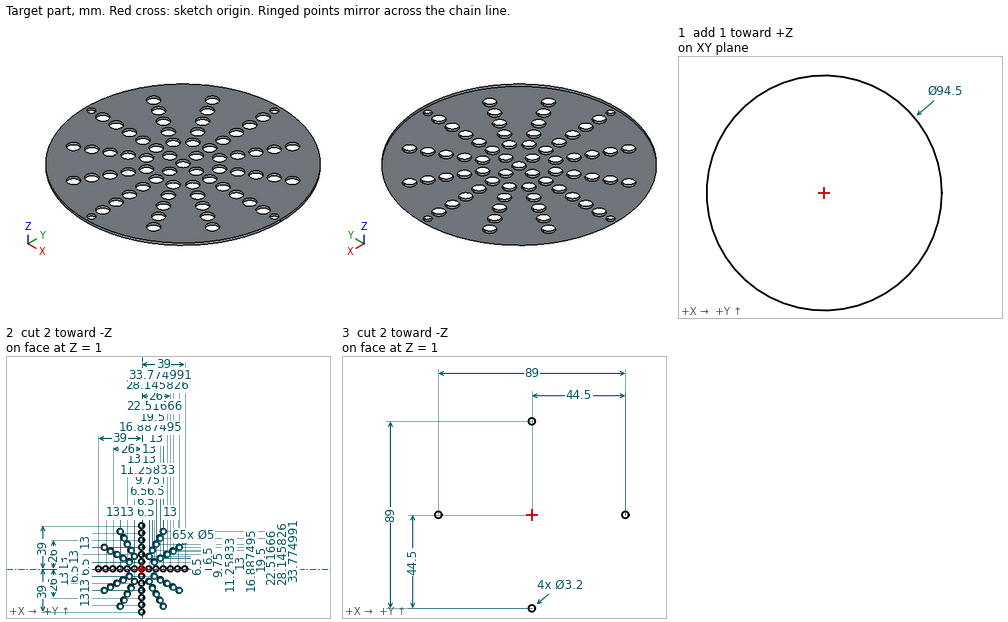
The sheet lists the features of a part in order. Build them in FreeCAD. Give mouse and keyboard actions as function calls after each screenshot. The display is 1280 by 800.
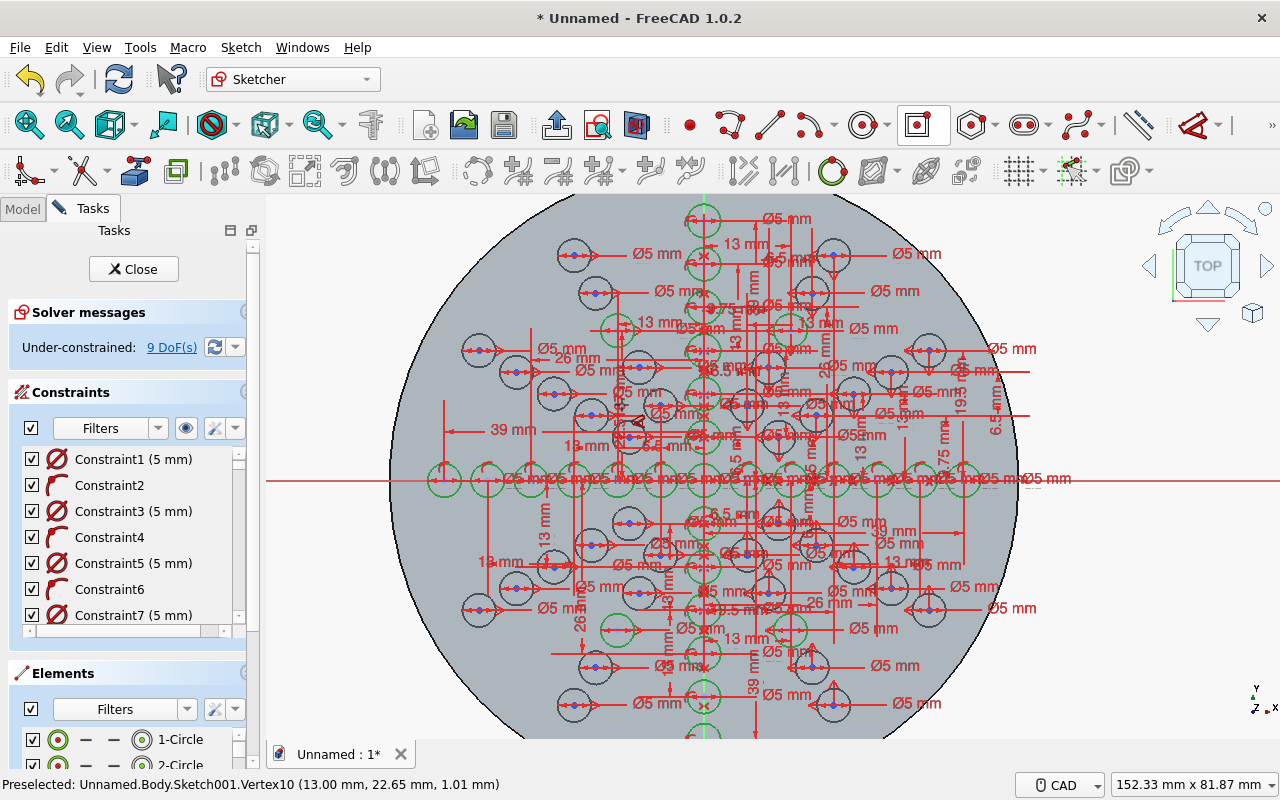
click(747, 406)
click(781, 443)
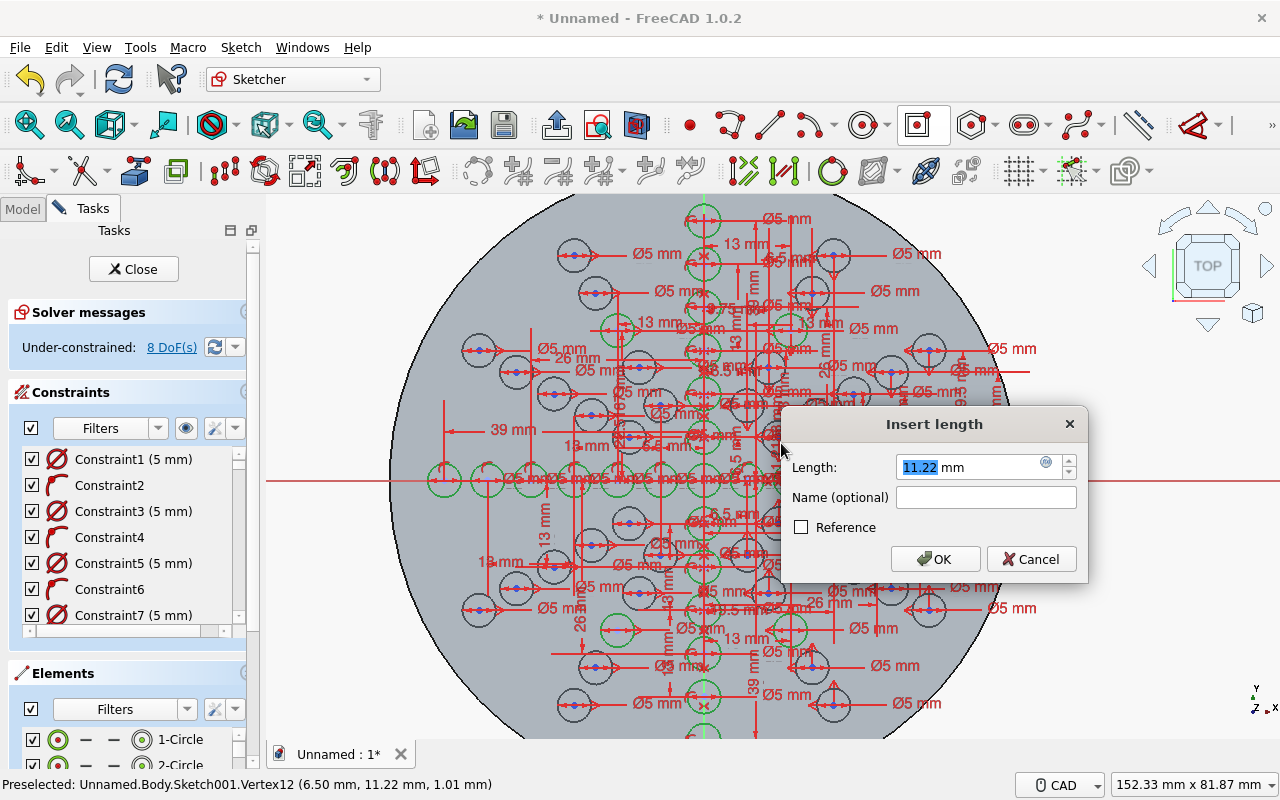
text(11.25833)
key(Return)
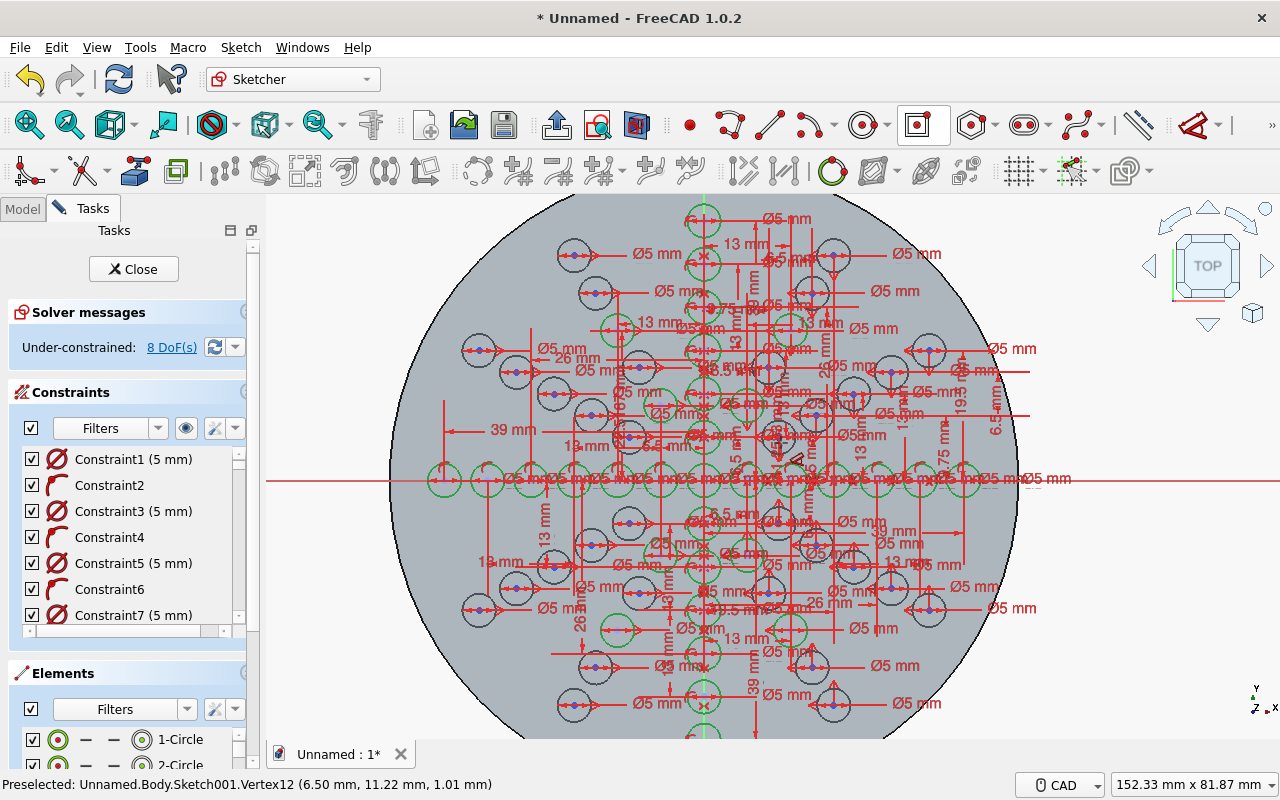
click(854, 394)
click(779, 563)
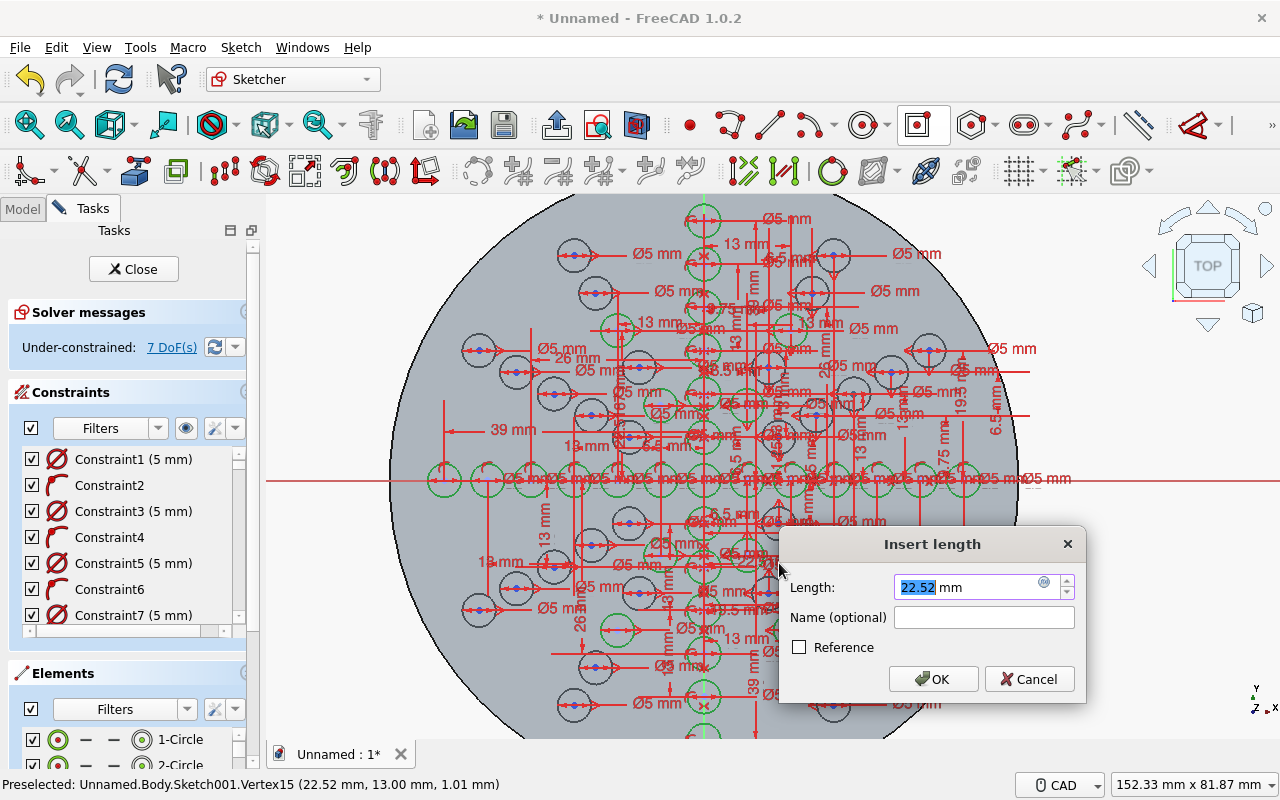
text(22.51666)
key(Return)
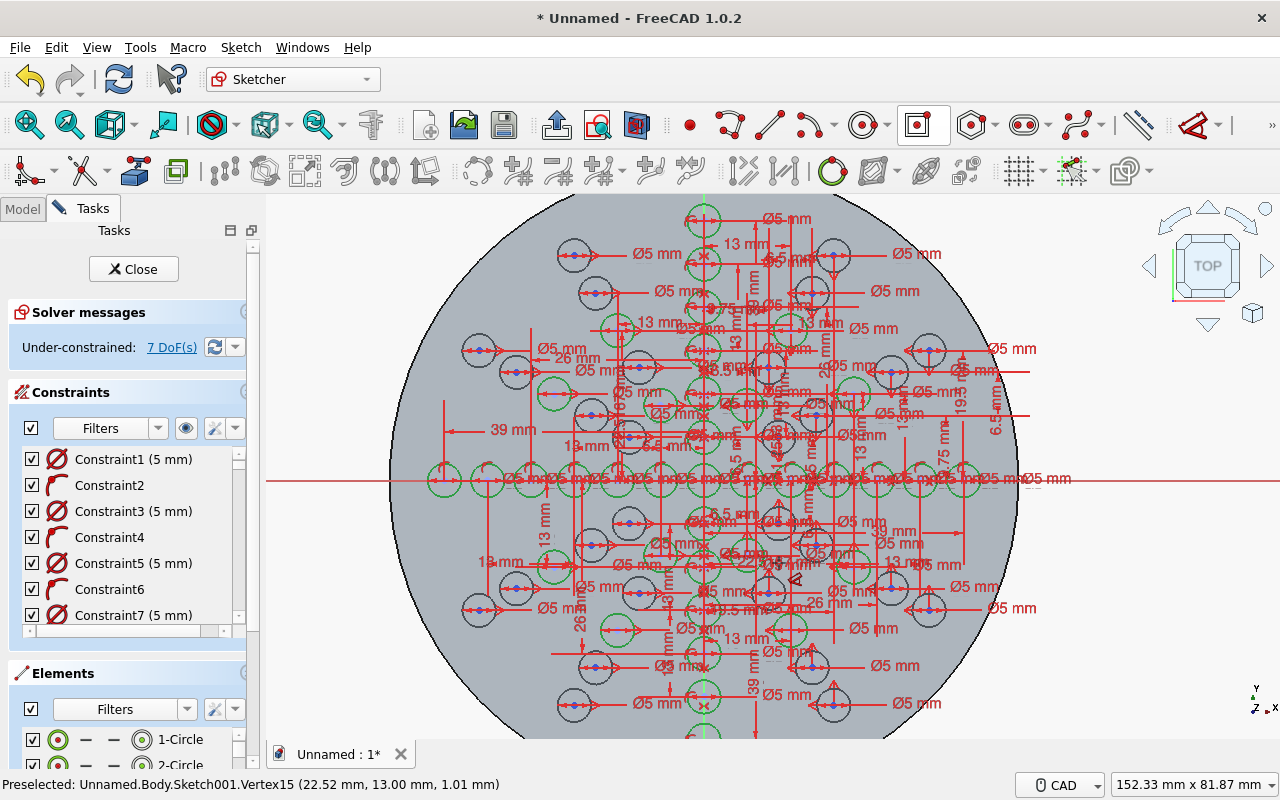
click(779, 437)
click(741, 403)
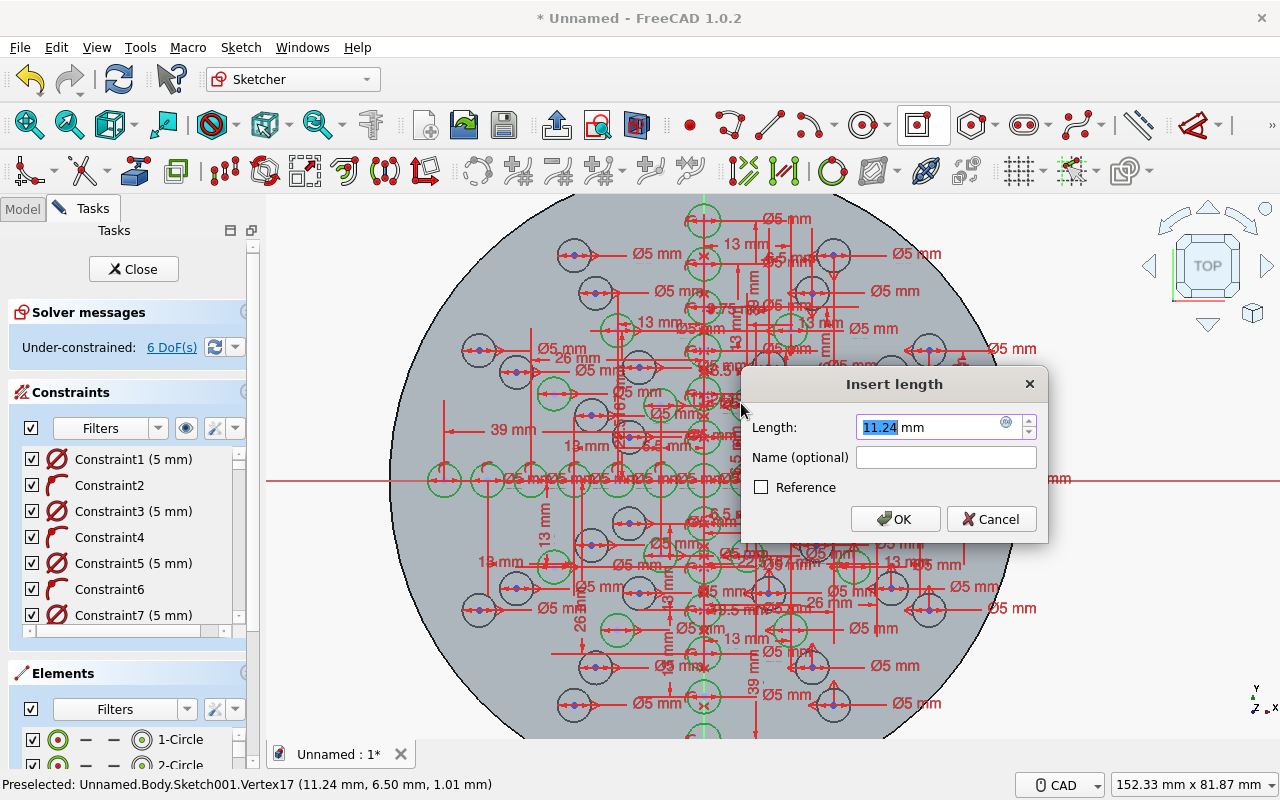
text(11.25833)
key(Return)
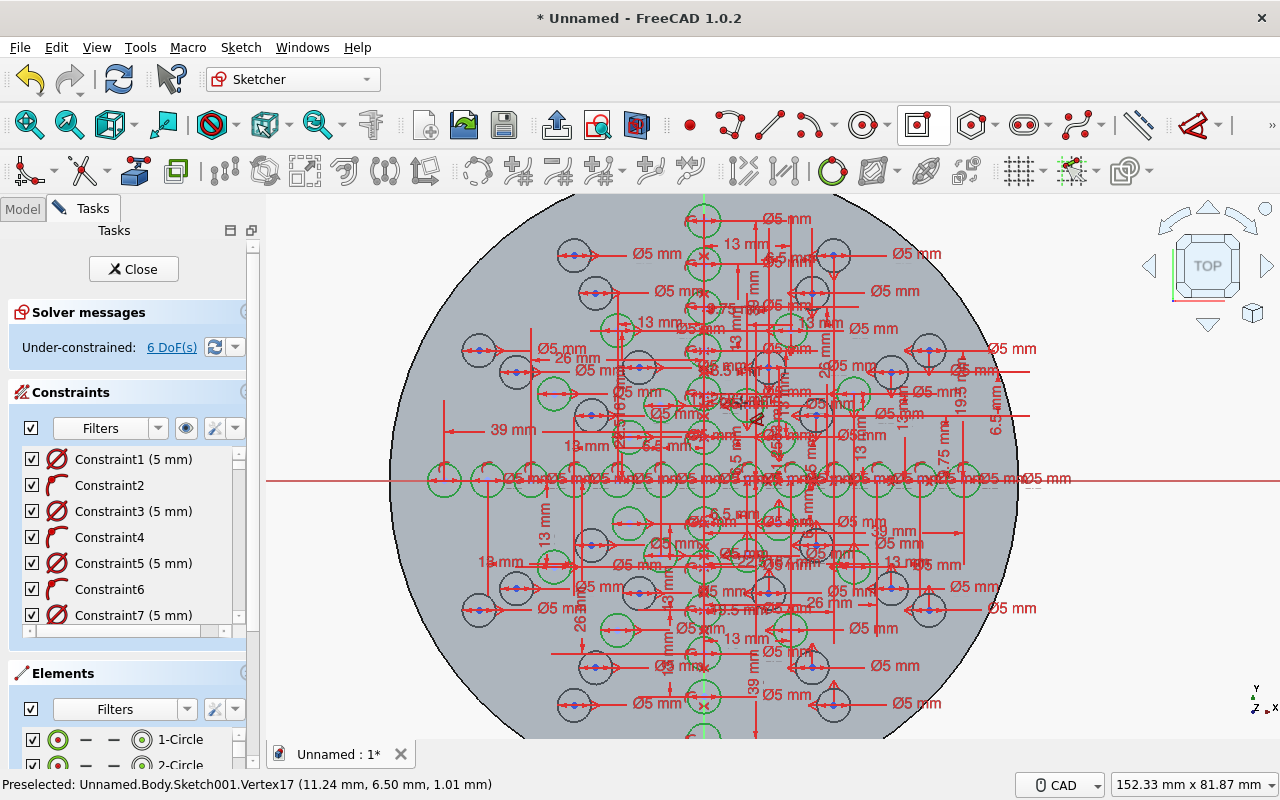
click(834, 256)
click(868, 289)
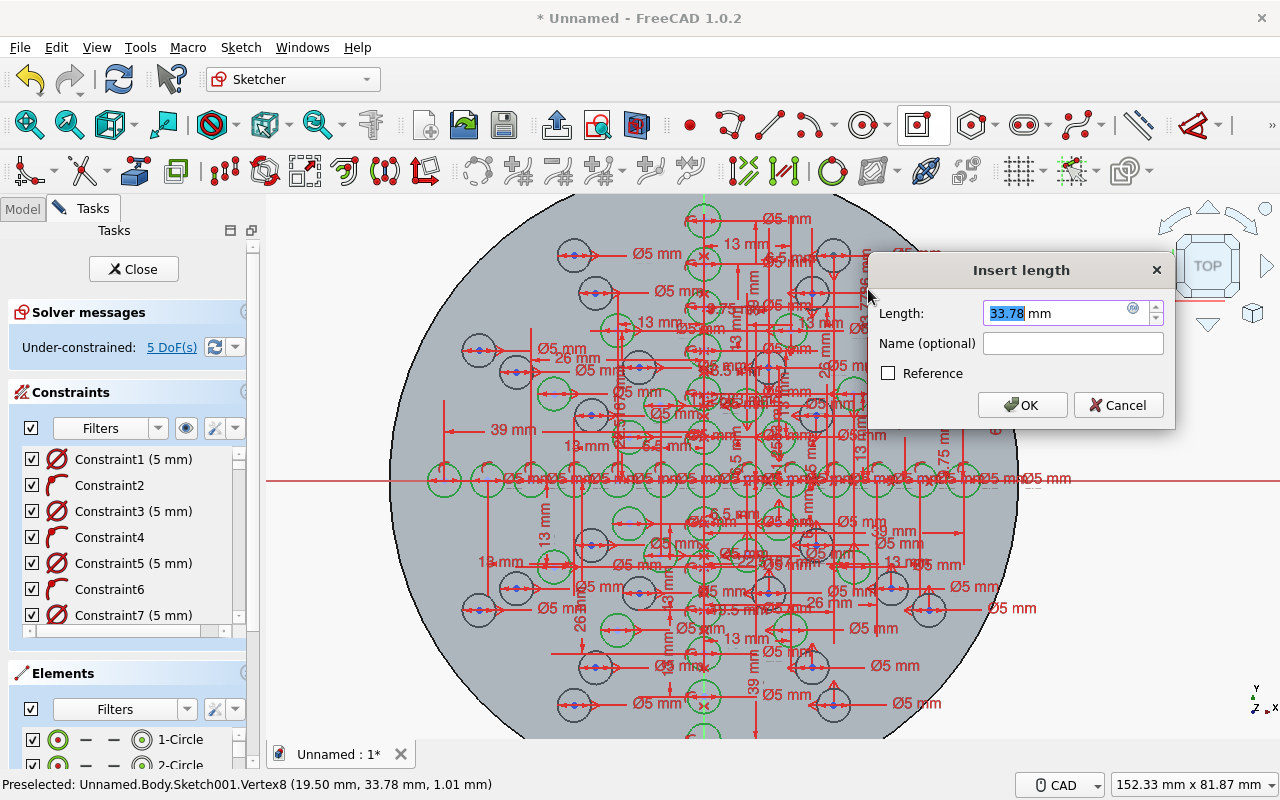
text(33.774991)
key(Return)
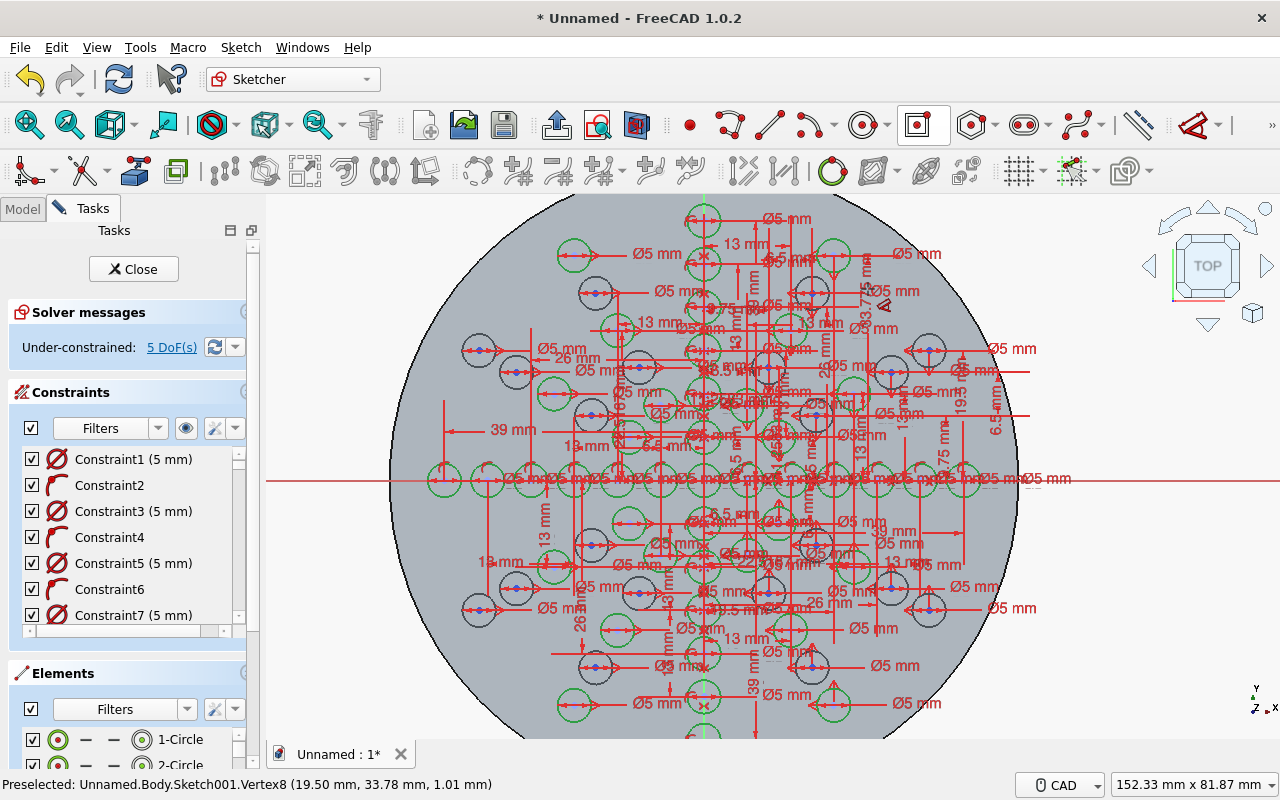
click(812, 293)
click(894, 321)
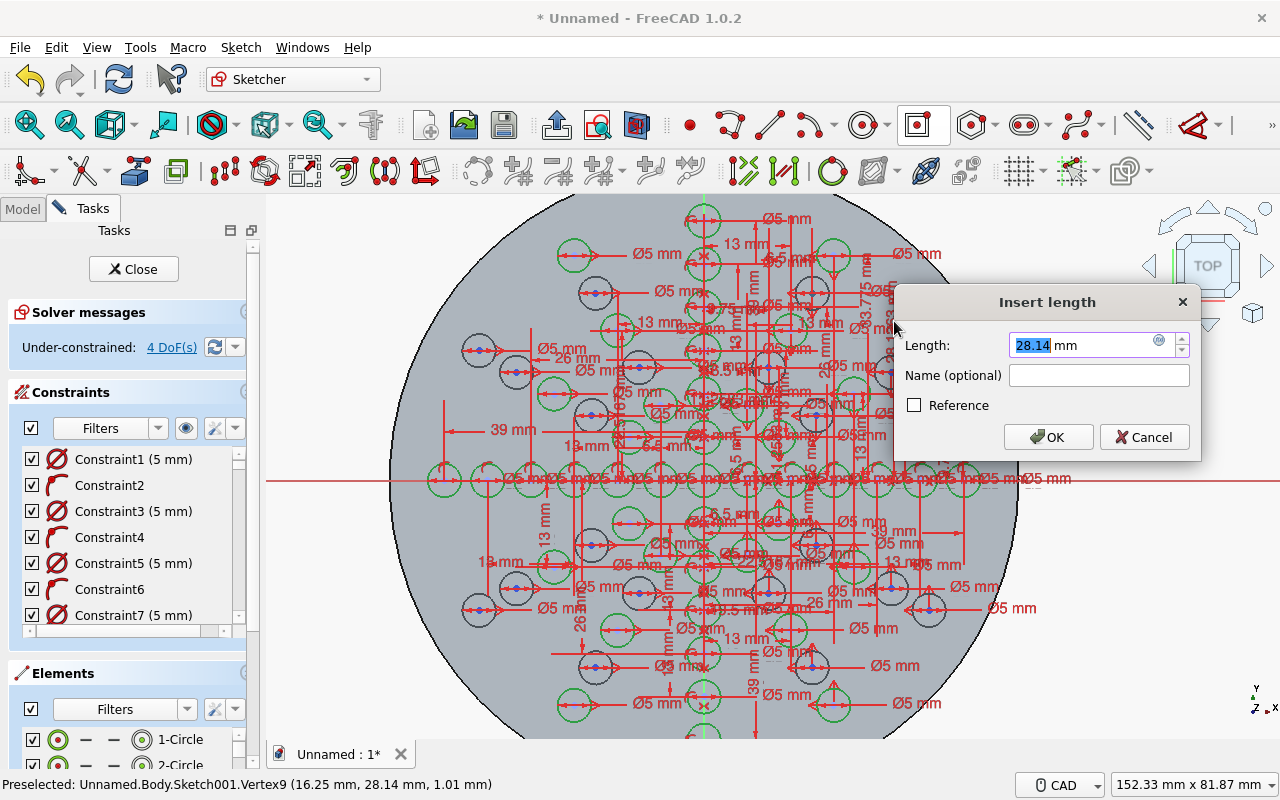
text(28.145826)
key(Return)